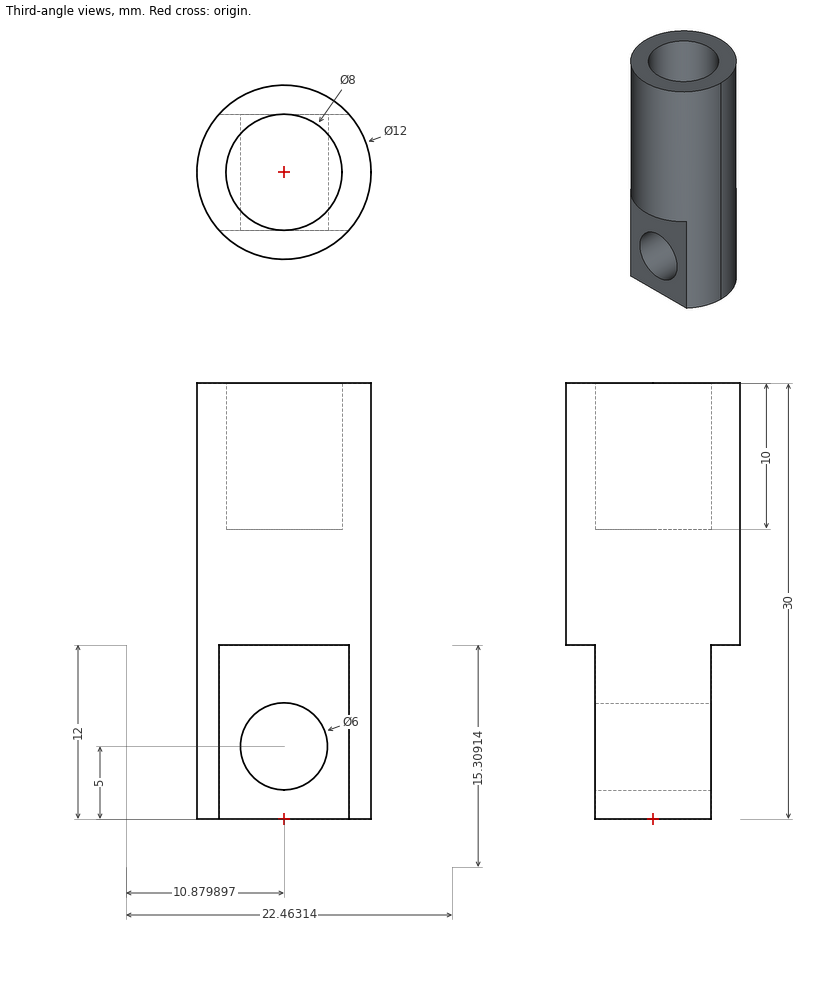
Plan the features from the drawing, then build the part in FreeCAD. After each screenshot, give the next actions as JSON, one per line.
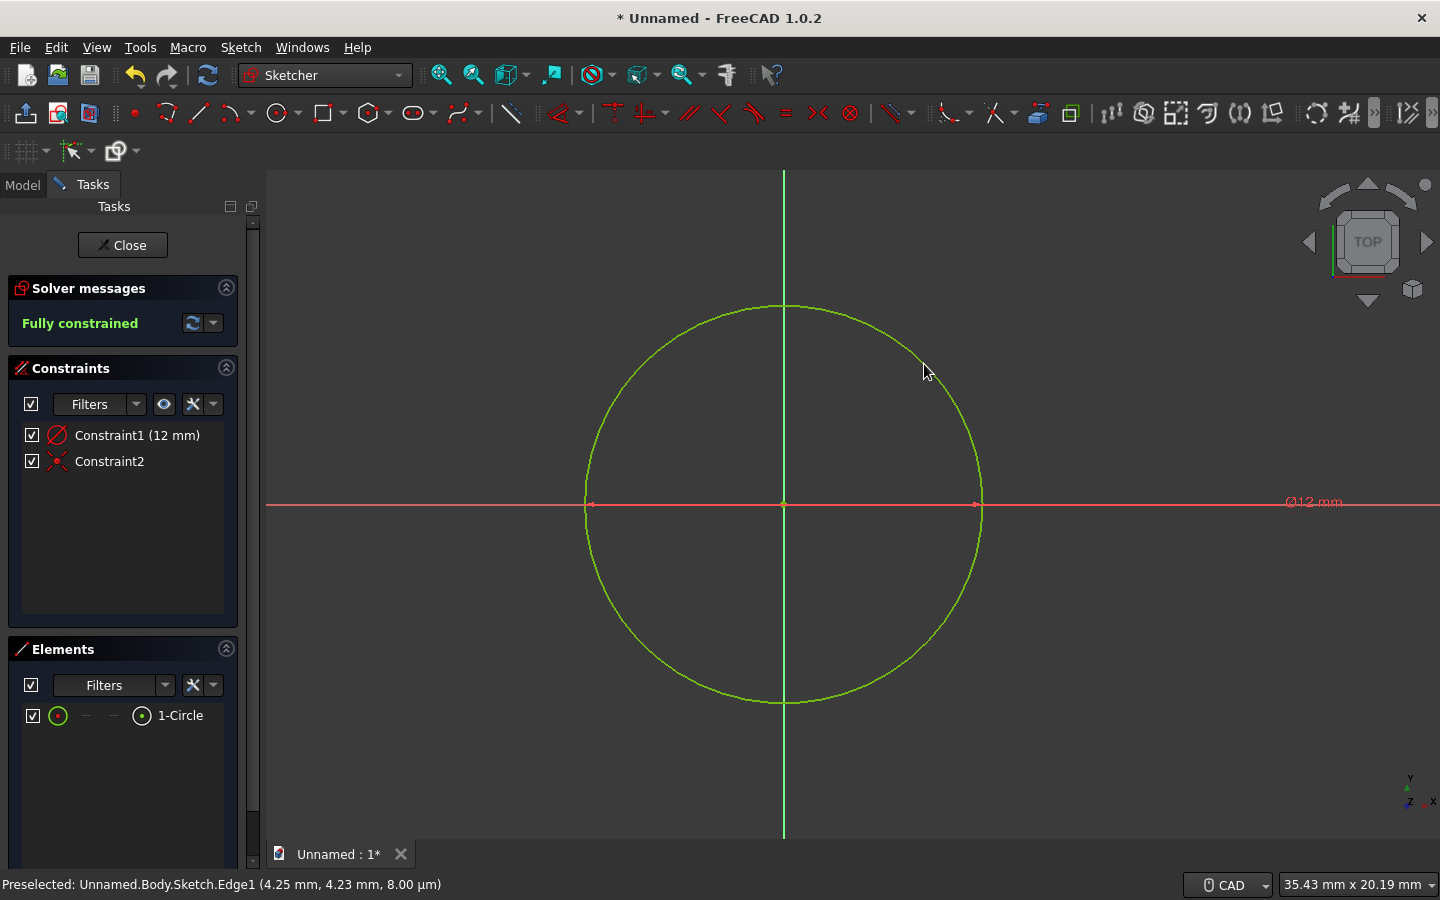
{"action": "left_click", "coordinate": [123, 245]}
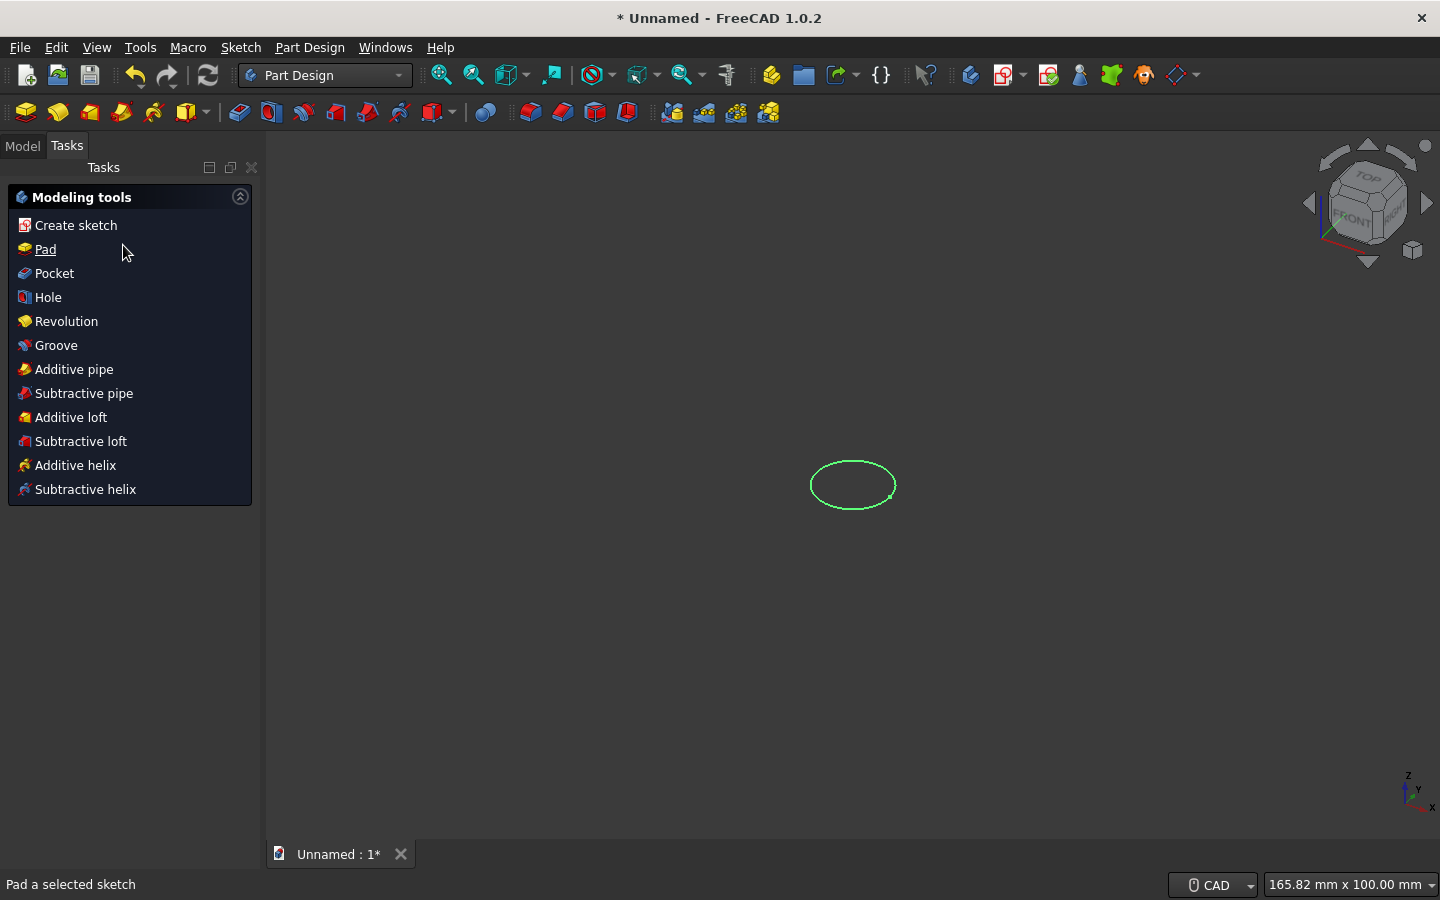
{"action": "left_click", "coordinate": [26, 112]}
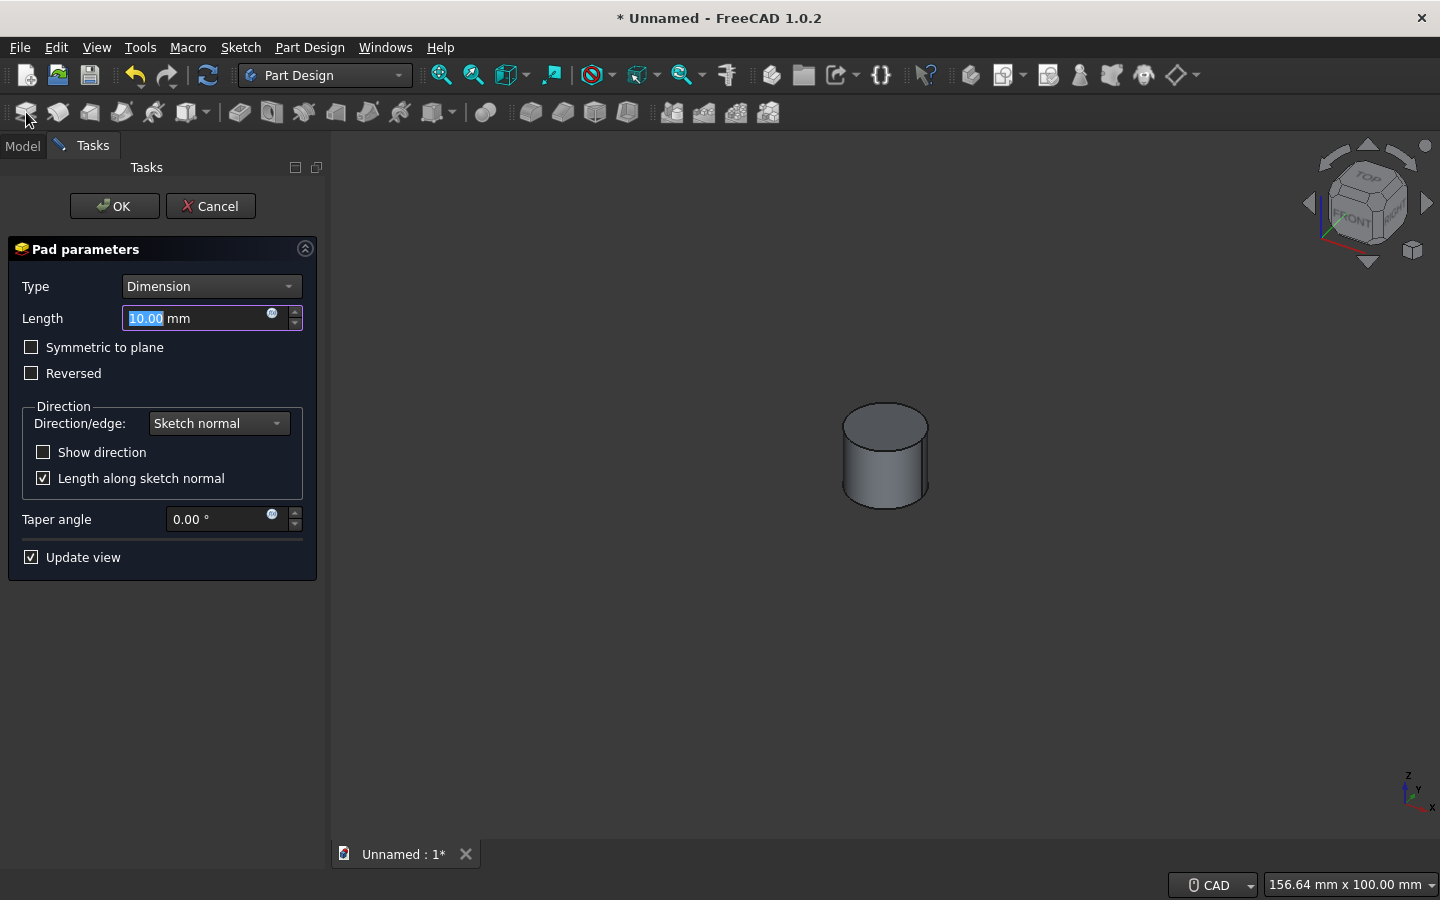
{"action": "type", "text": "30"}
{"action": "key", "text": "Tab"}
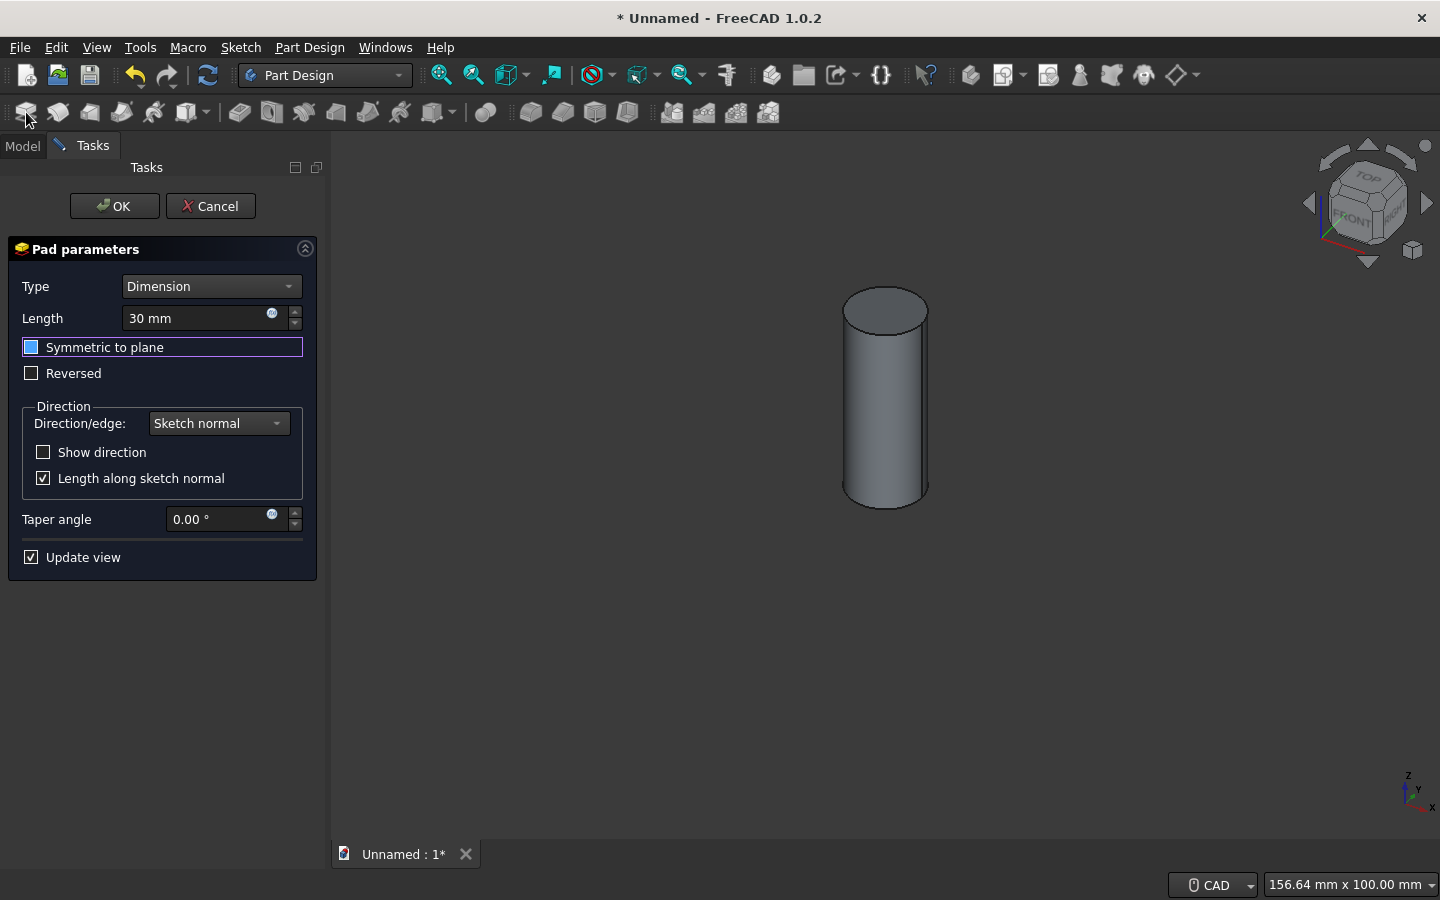
{"action": "left_click", "coordinate": [115, 206]}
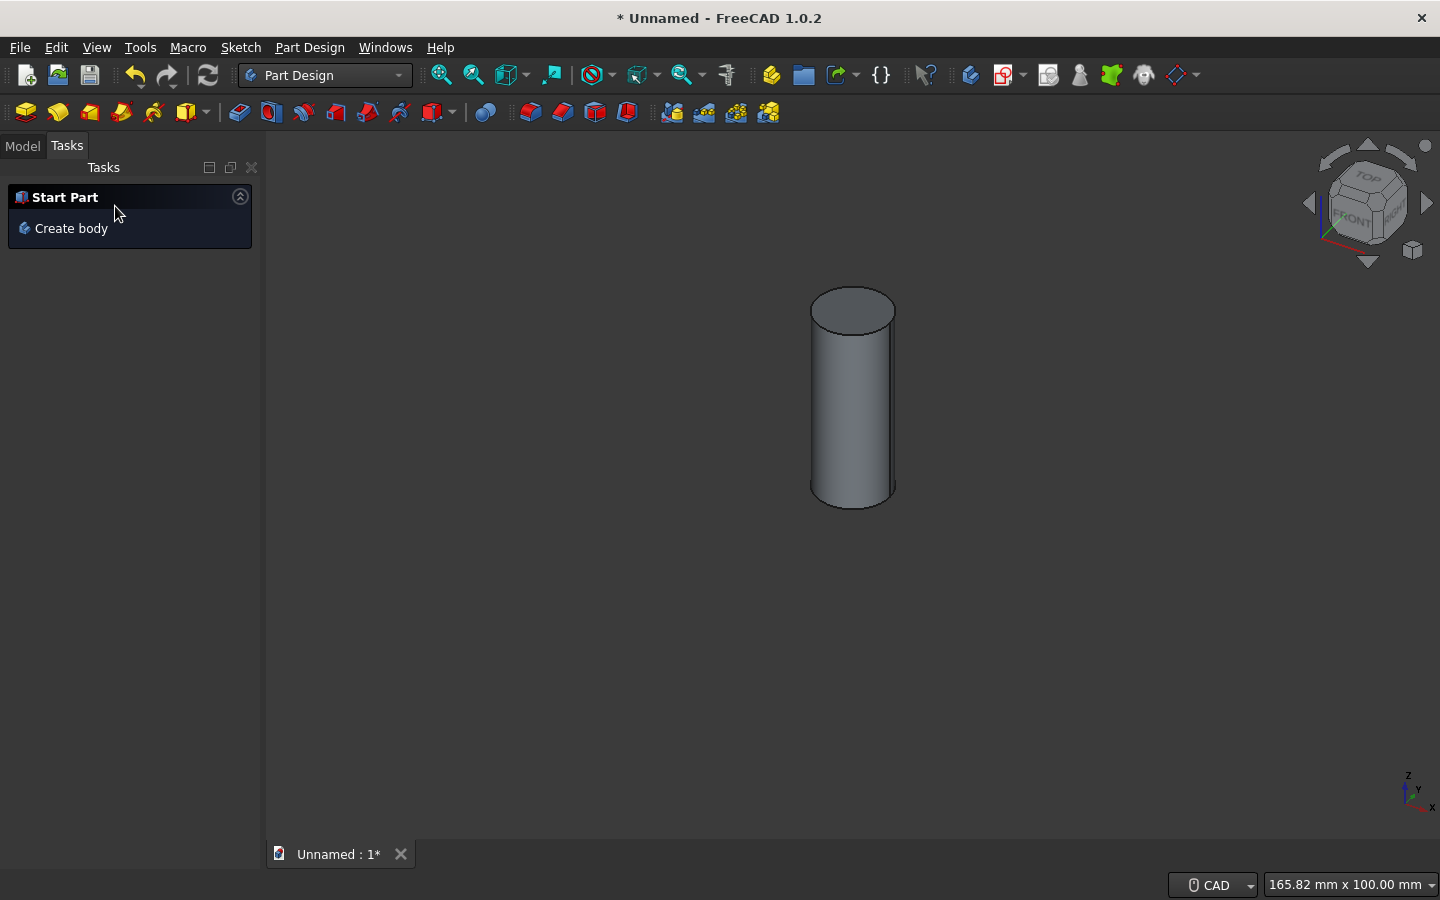
{"action": "left_click", "coordinate": [442, 76]}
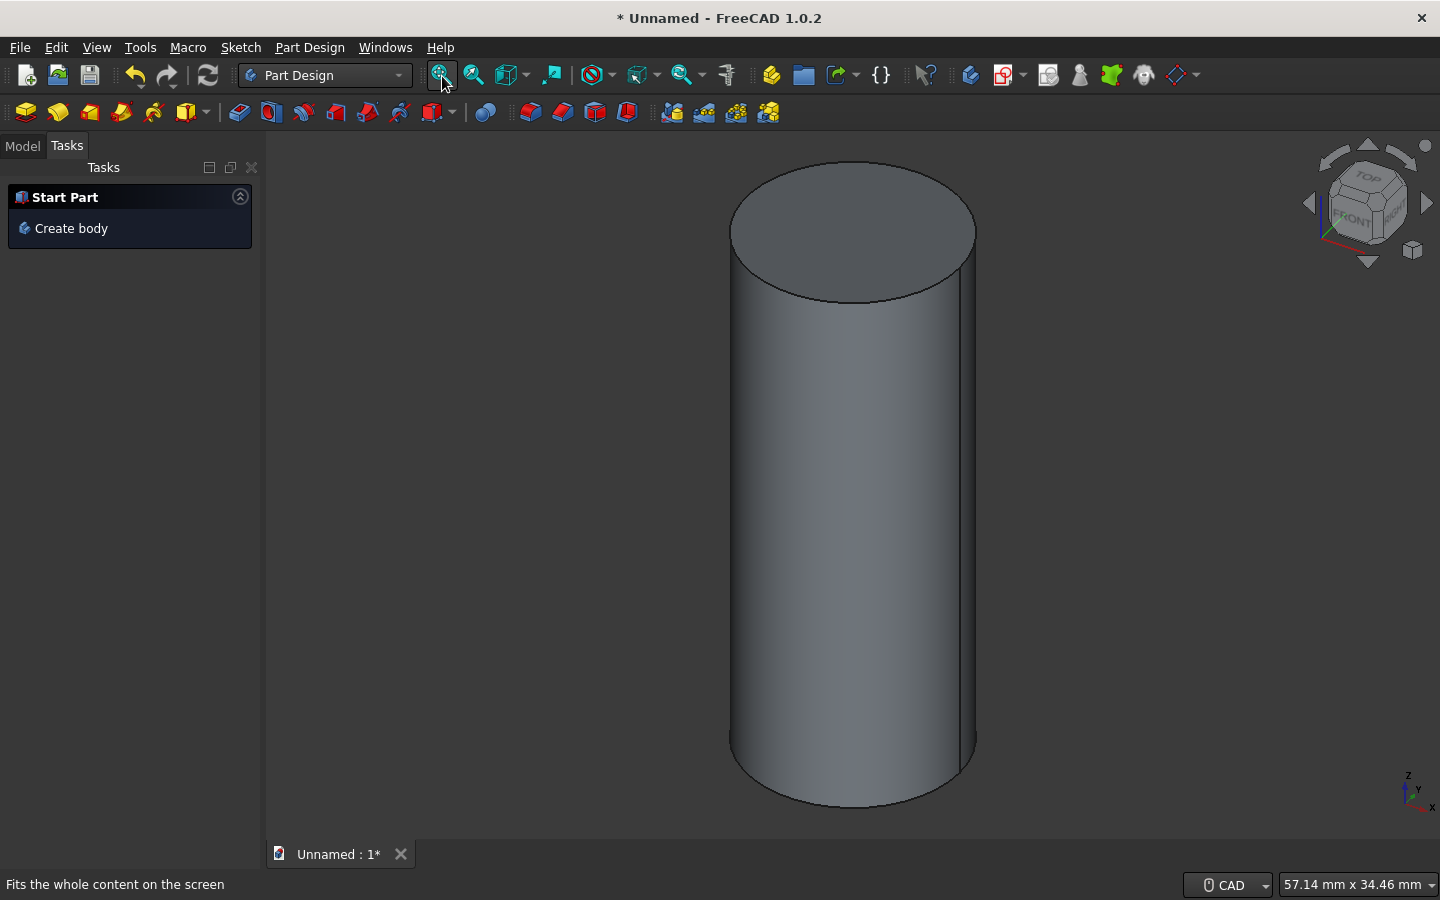
{"action": "left_click", "coordinate": [23, 145]}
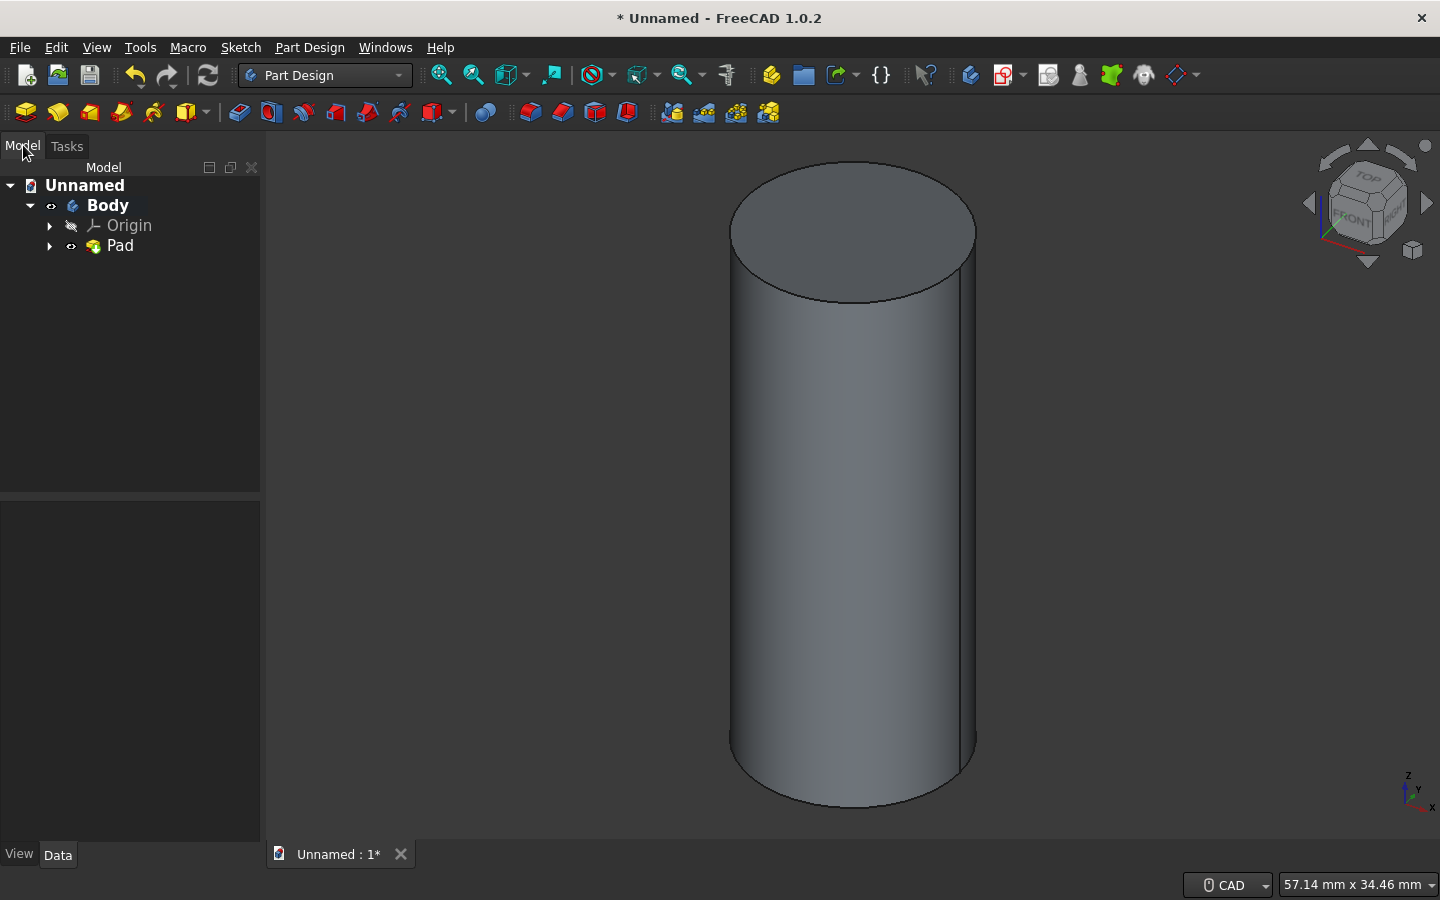
{"action": "left_click", "coordinate": [50, 226]}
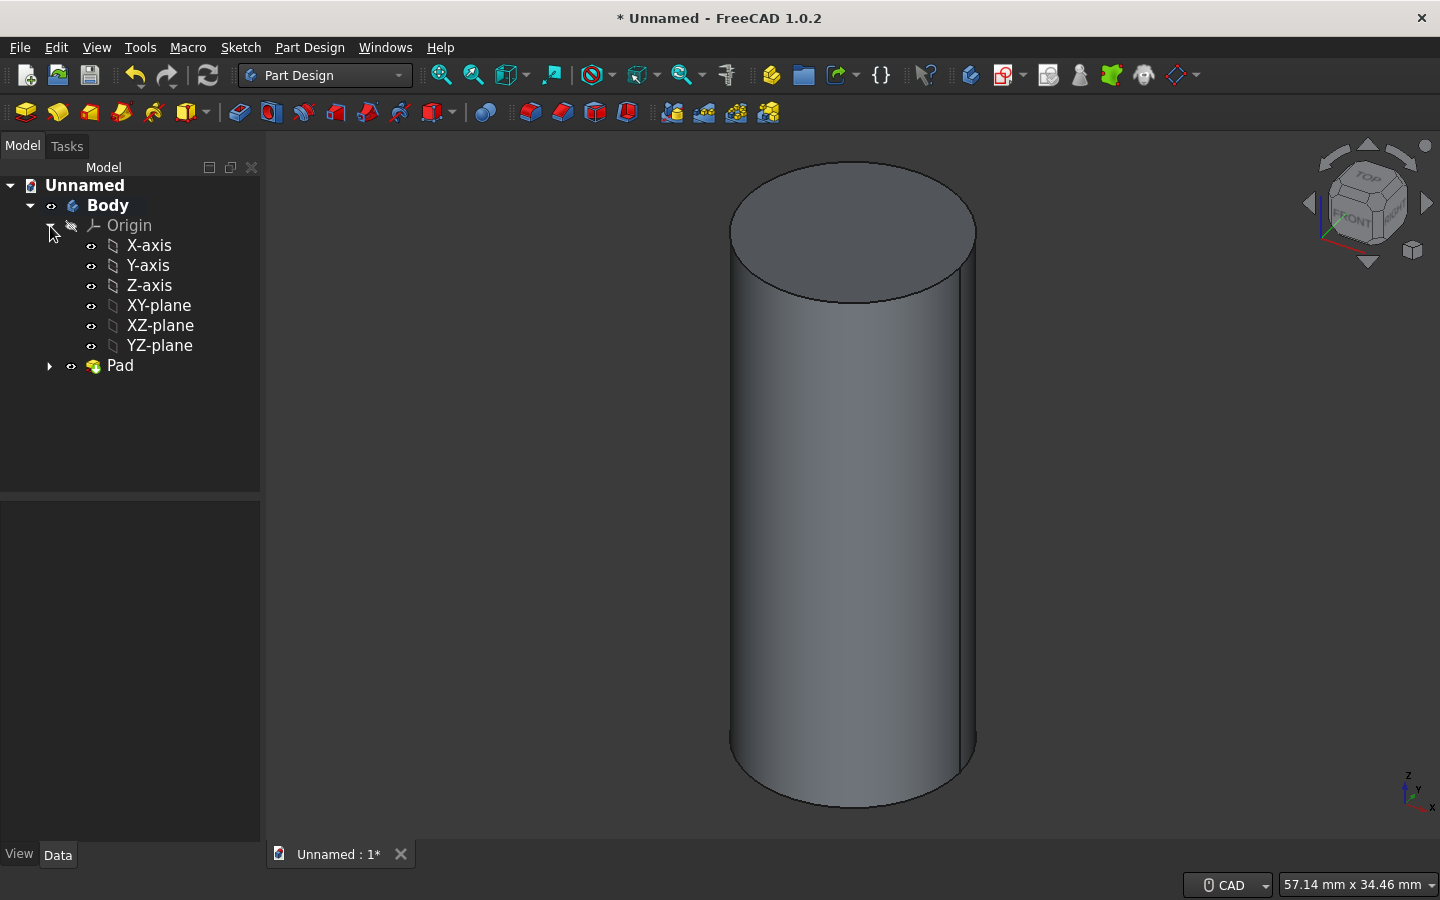
{"action": "left_click", "coordinate": [136, 326]}